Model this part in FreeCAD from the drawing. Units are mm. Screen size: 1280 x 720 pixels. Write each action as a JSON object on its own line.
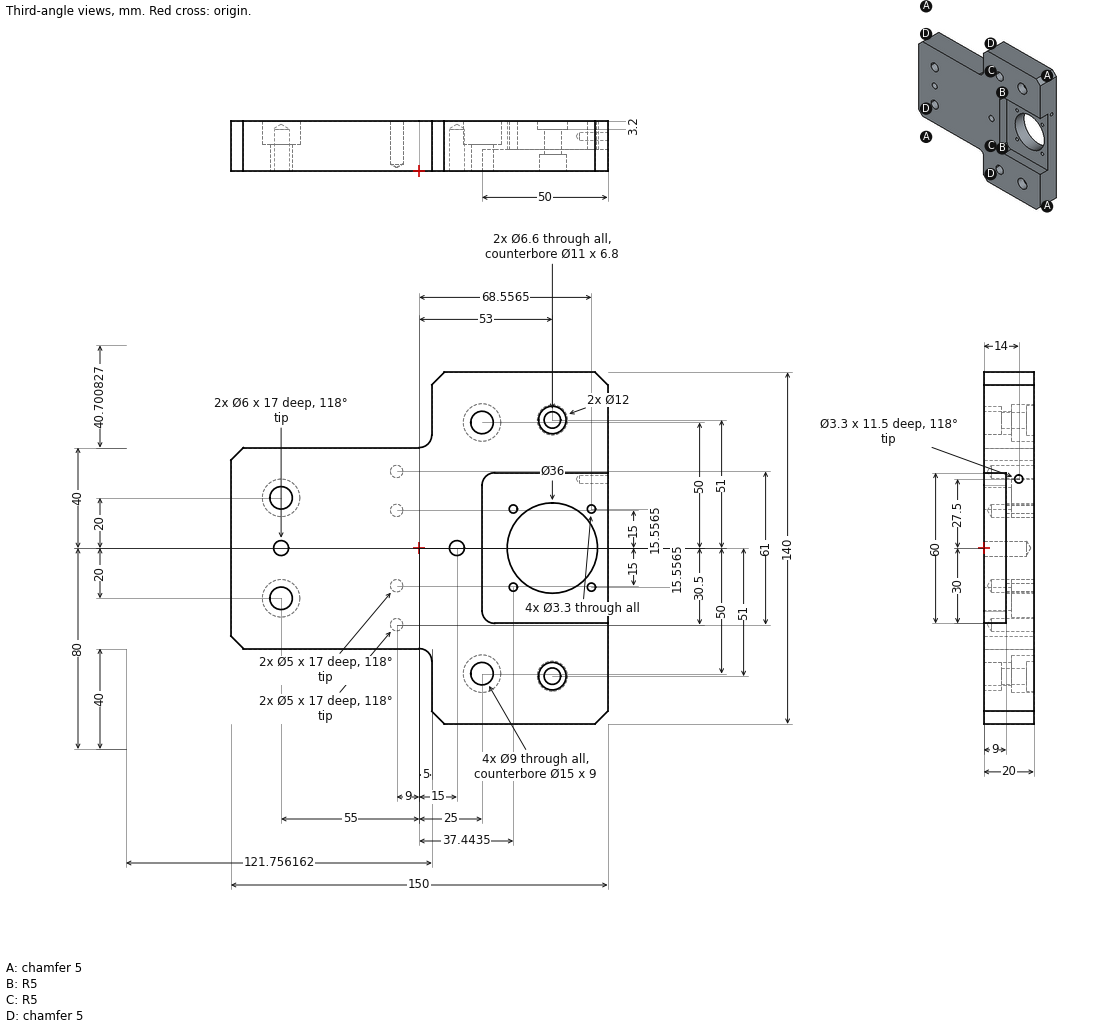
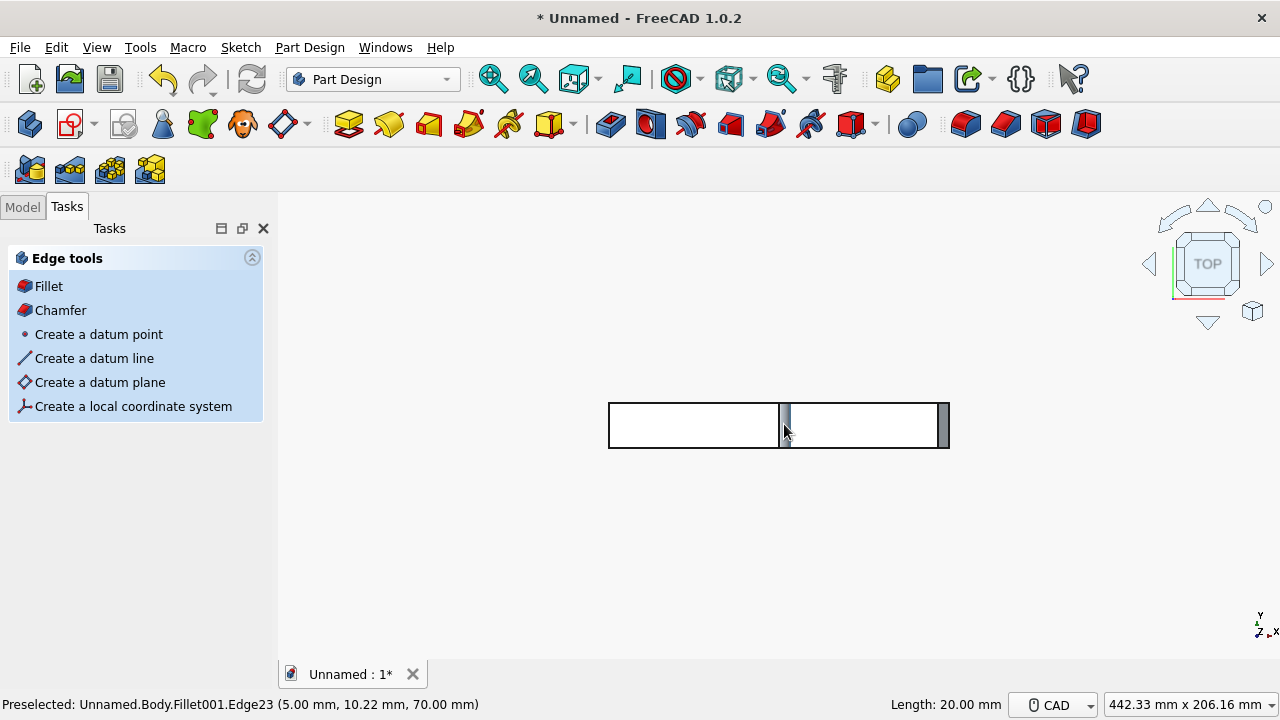
{"action": "left_click", "coordinate": [609, 424], "text": "ctrl"}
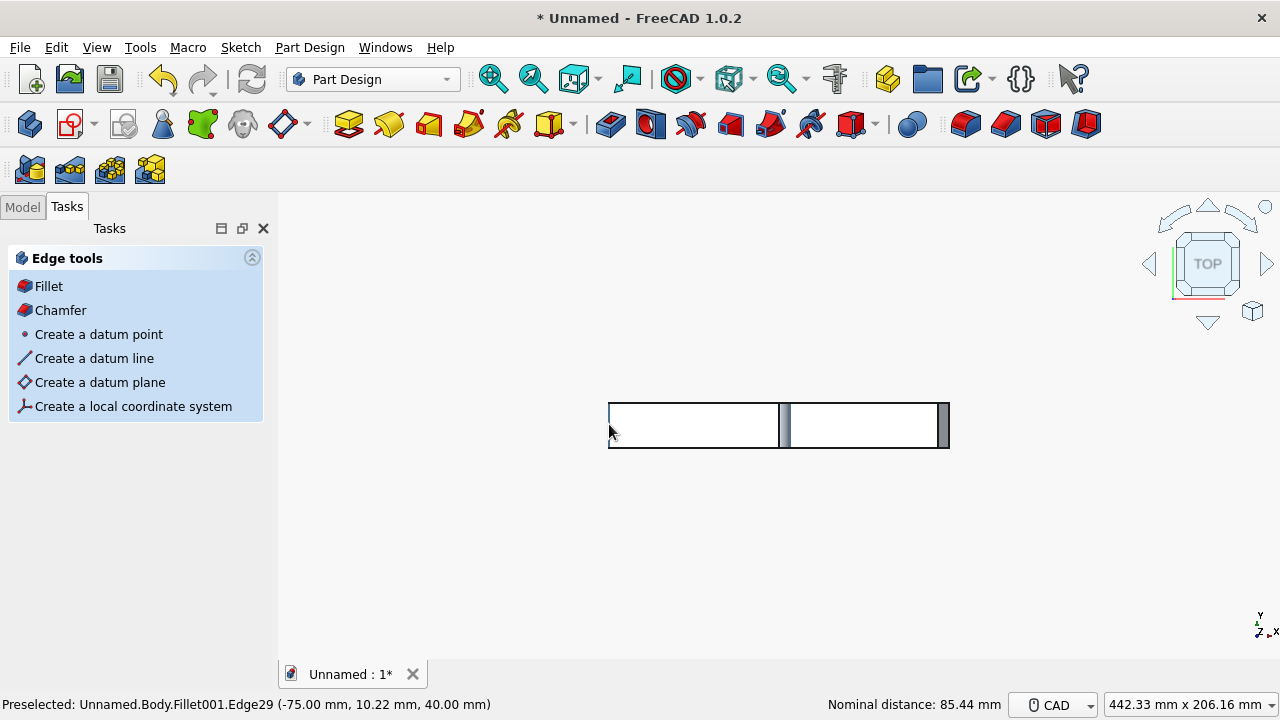
{"action": "key", "text": "0"}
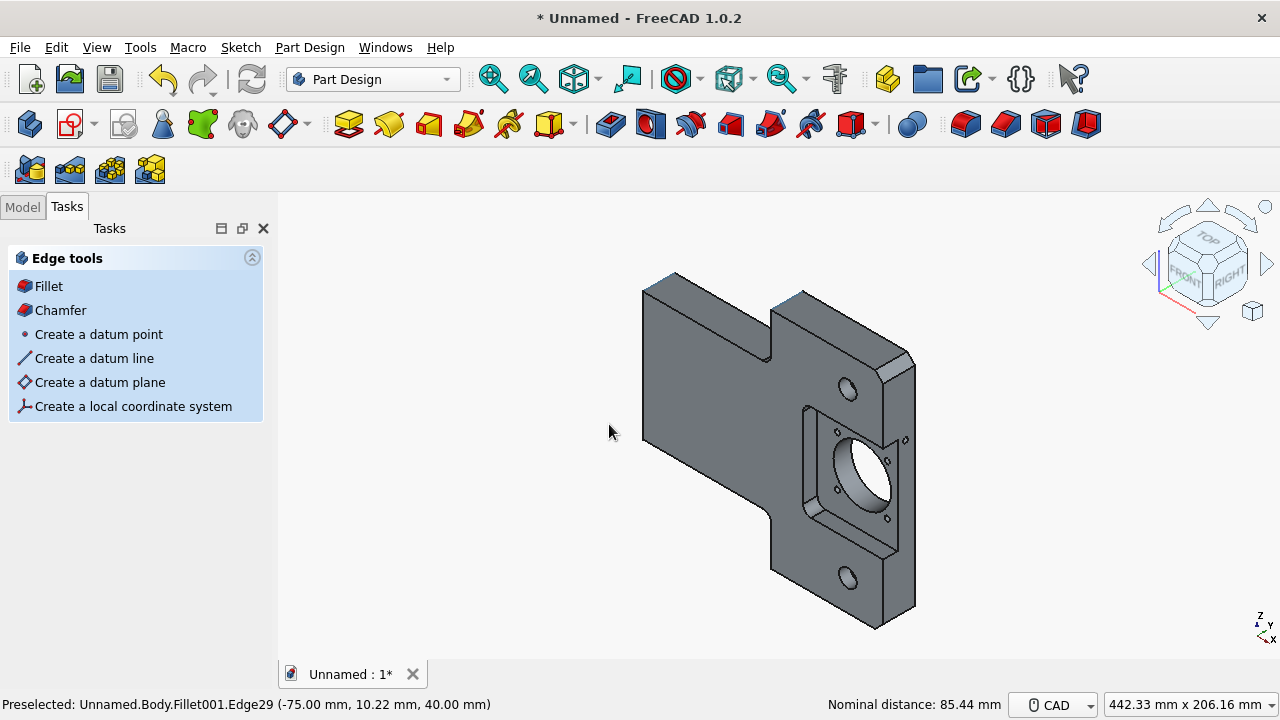
{"action": "key", "text": "1"}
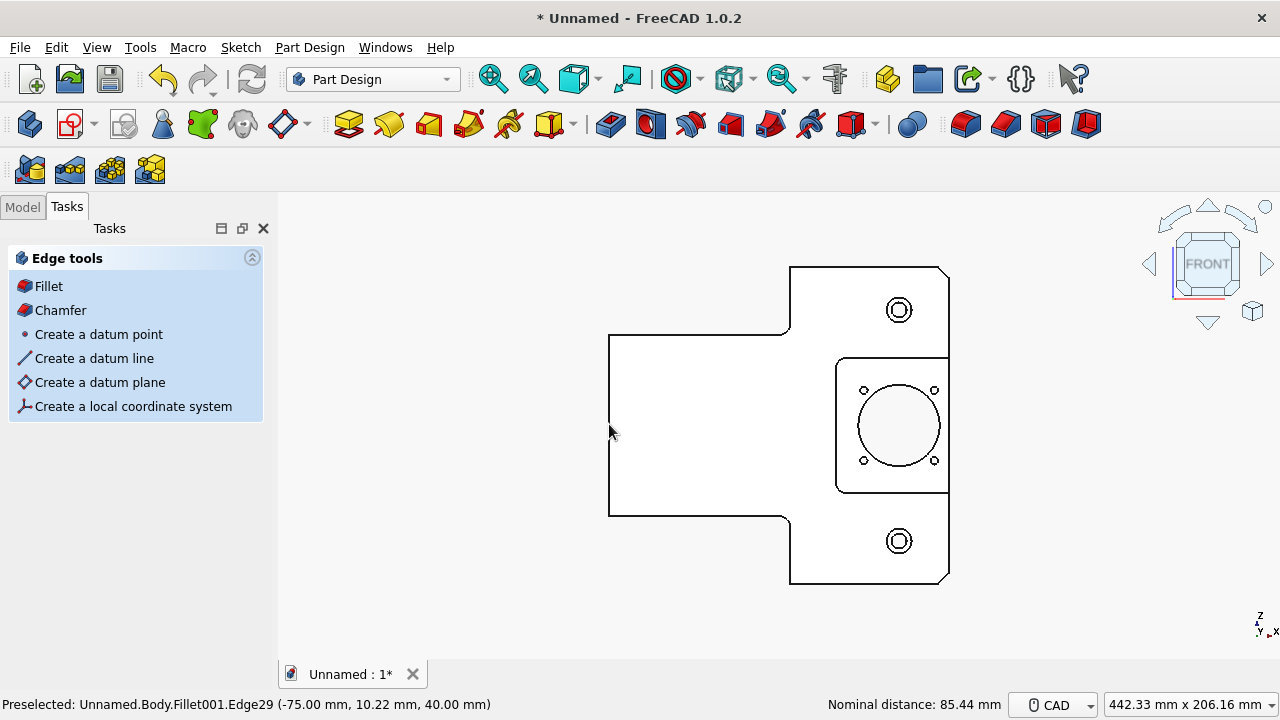
{"action": "key", "text": "3"}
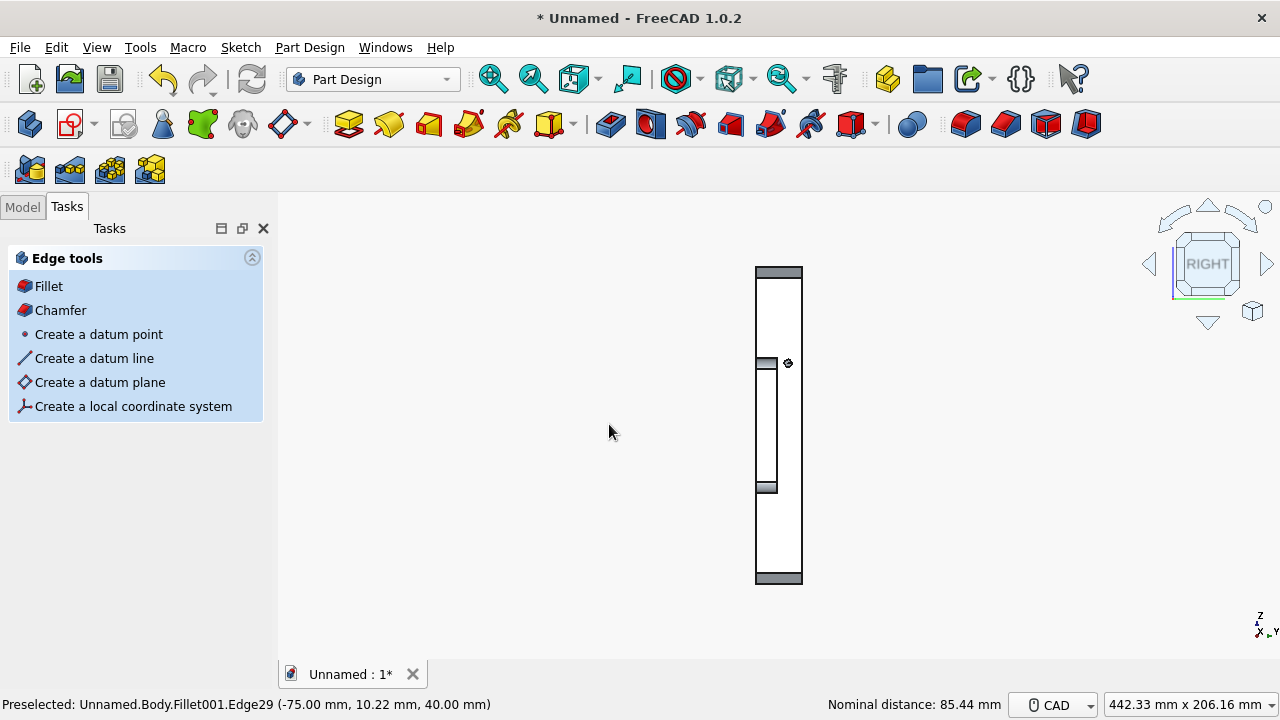
{"action": "key", "text": "5"}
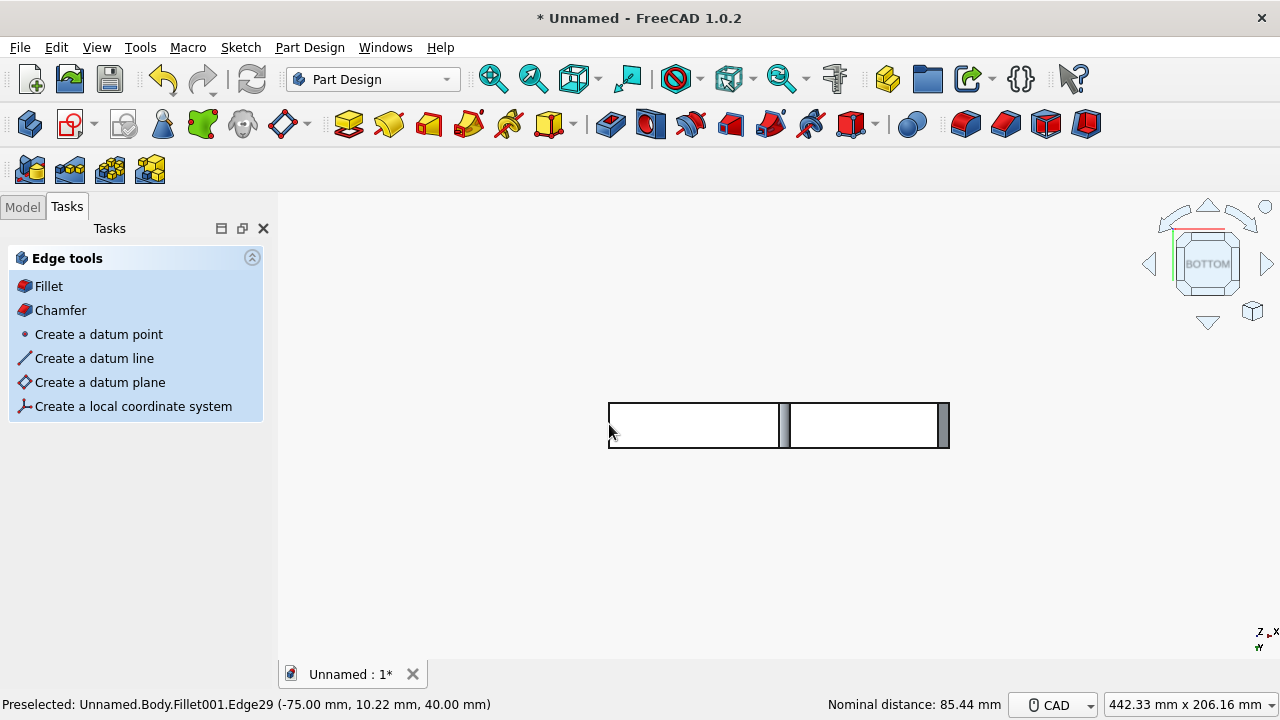
{"action": "left_click", "coordinate": [494, 80]}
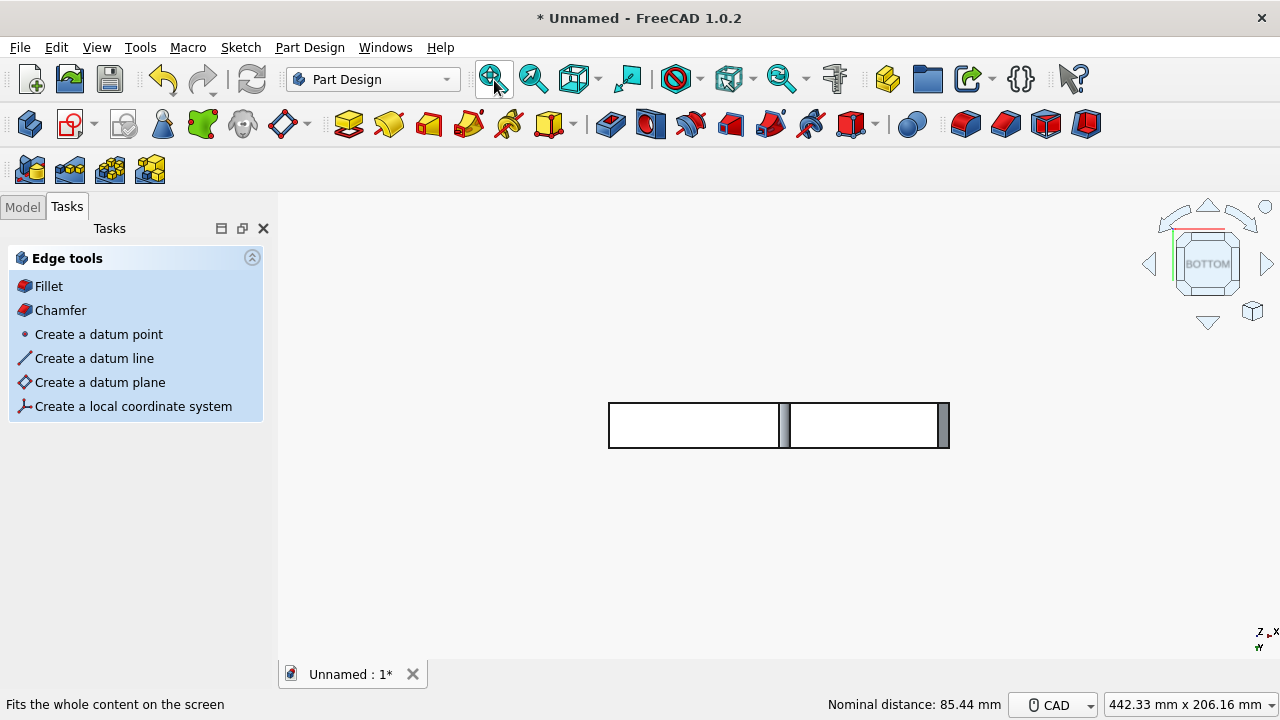
{"action": "left_click", "coordinate": [790, 424], "text": "ctrl"}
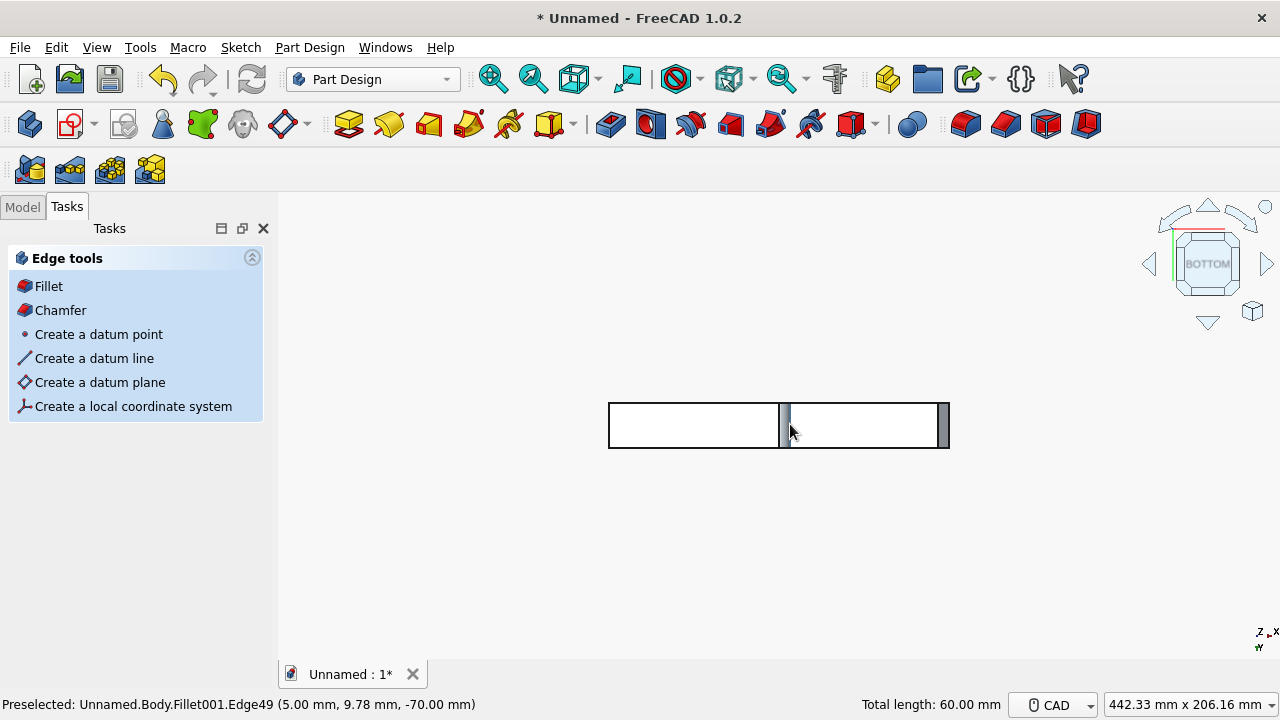
{"action": "left_click", "coordinate": [609, 424], "text": "ctrl"}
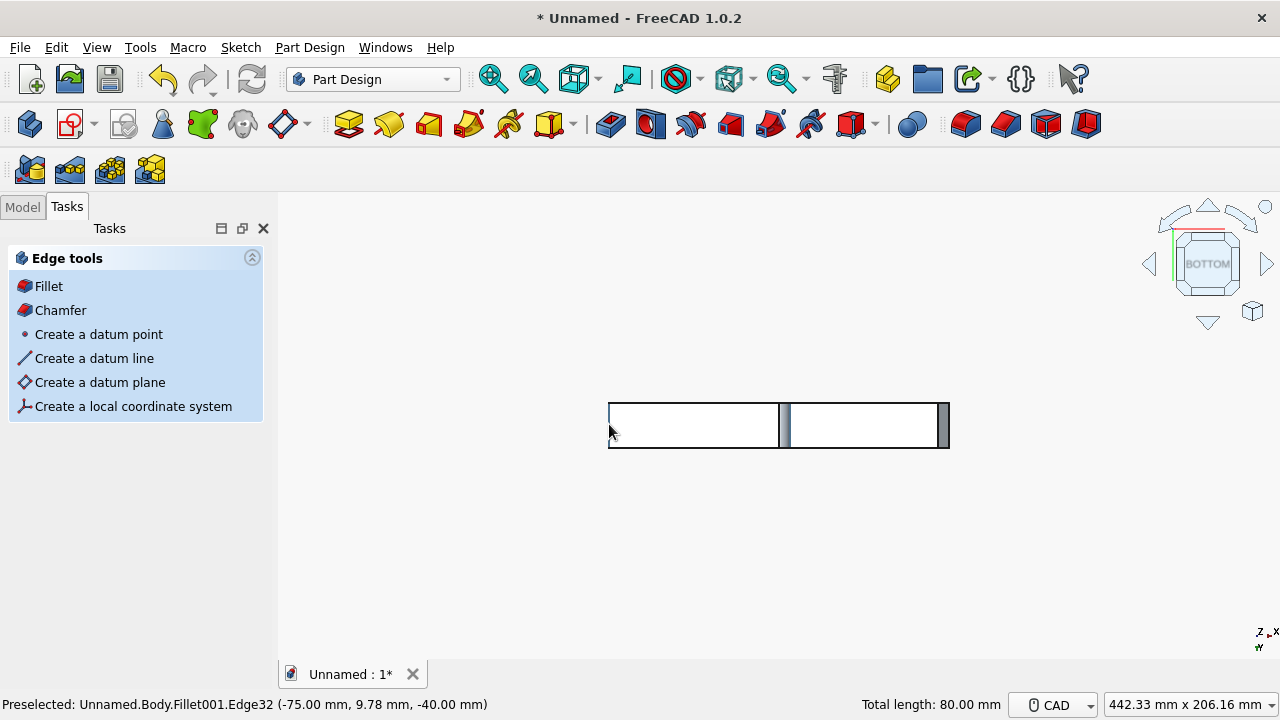
{"action": "left_click", "coordinate": [1006, 124]}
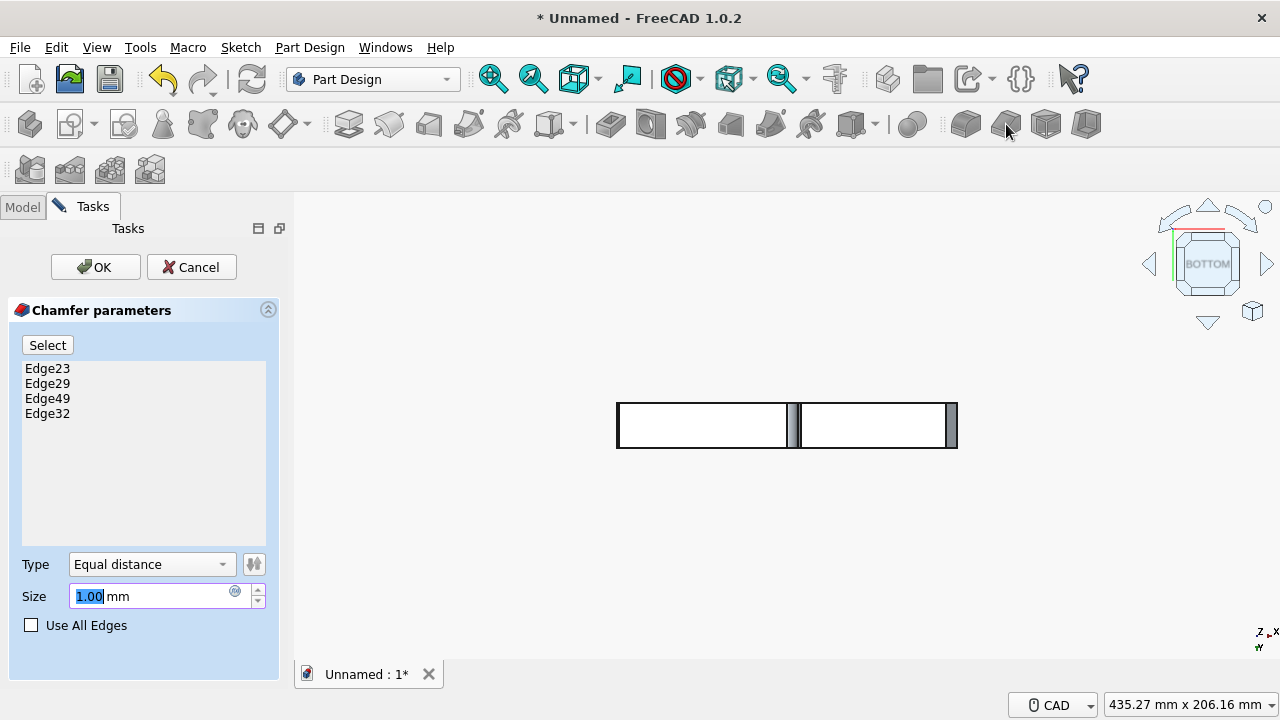
{"action": "type", "text": "5"}
{"action": "key", "text": "Tab"}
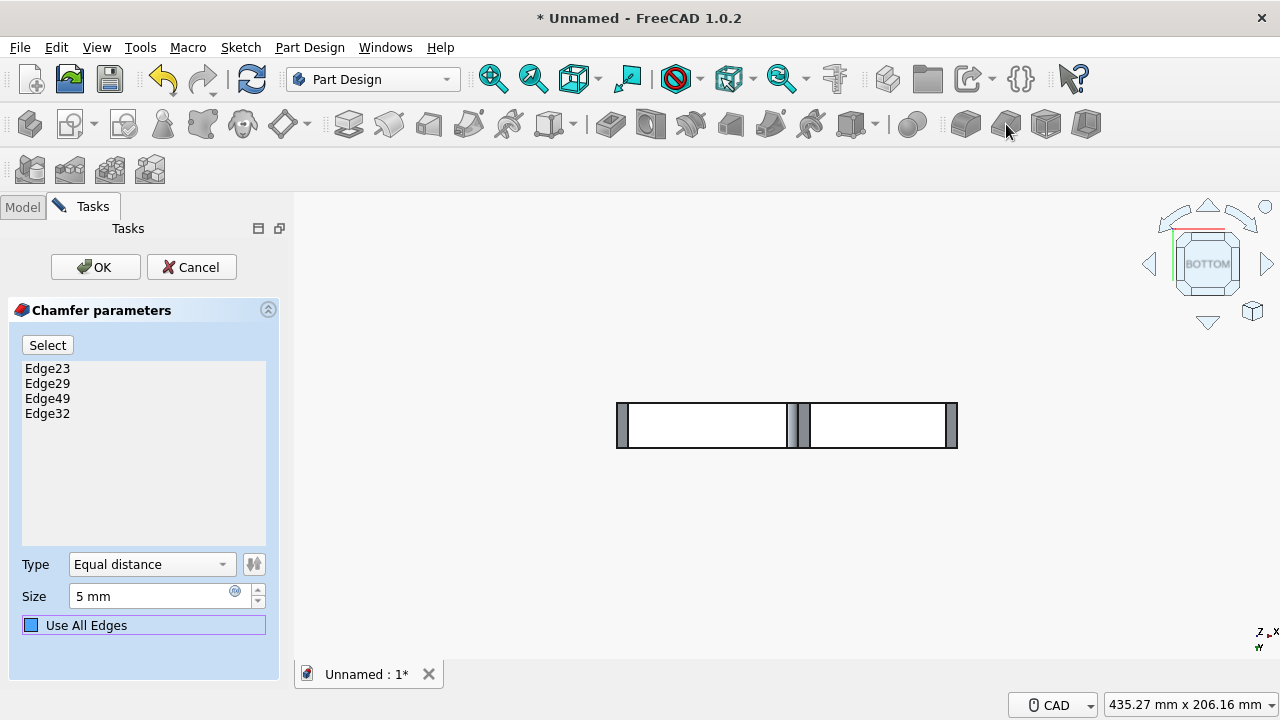
{"action": "left_click", "coordinate": [96, 267]}